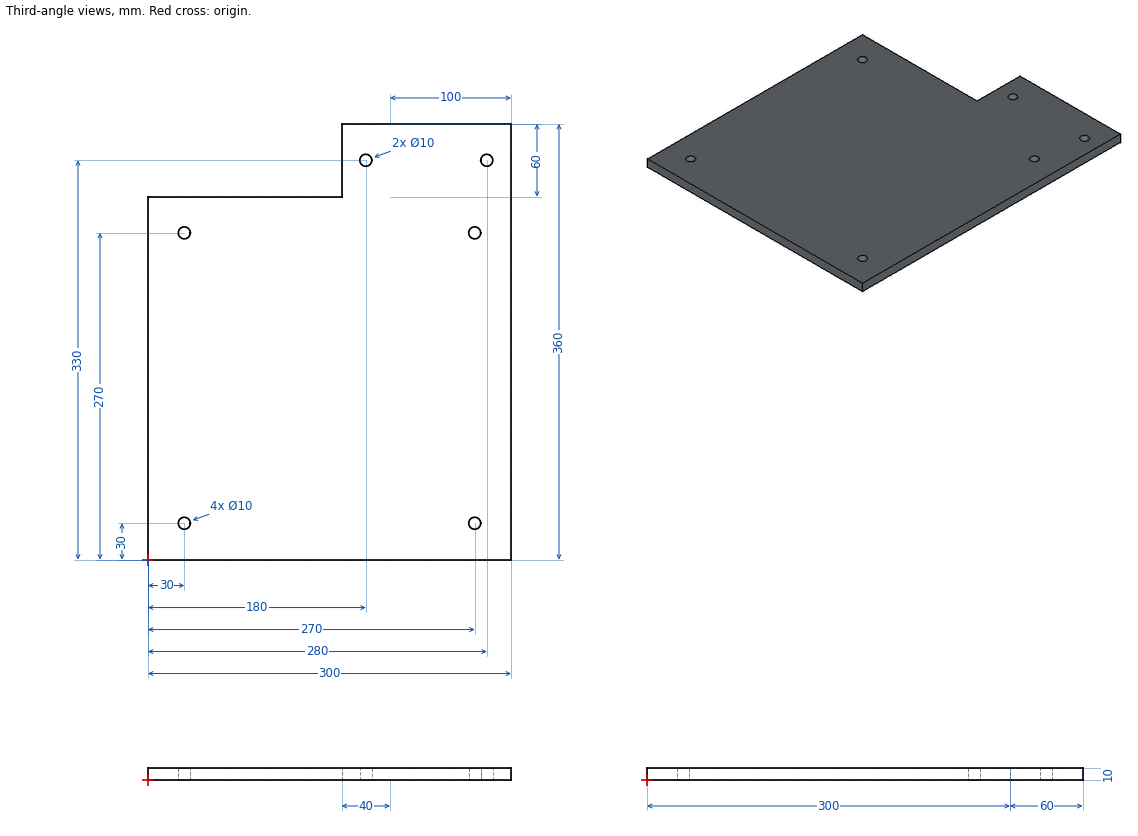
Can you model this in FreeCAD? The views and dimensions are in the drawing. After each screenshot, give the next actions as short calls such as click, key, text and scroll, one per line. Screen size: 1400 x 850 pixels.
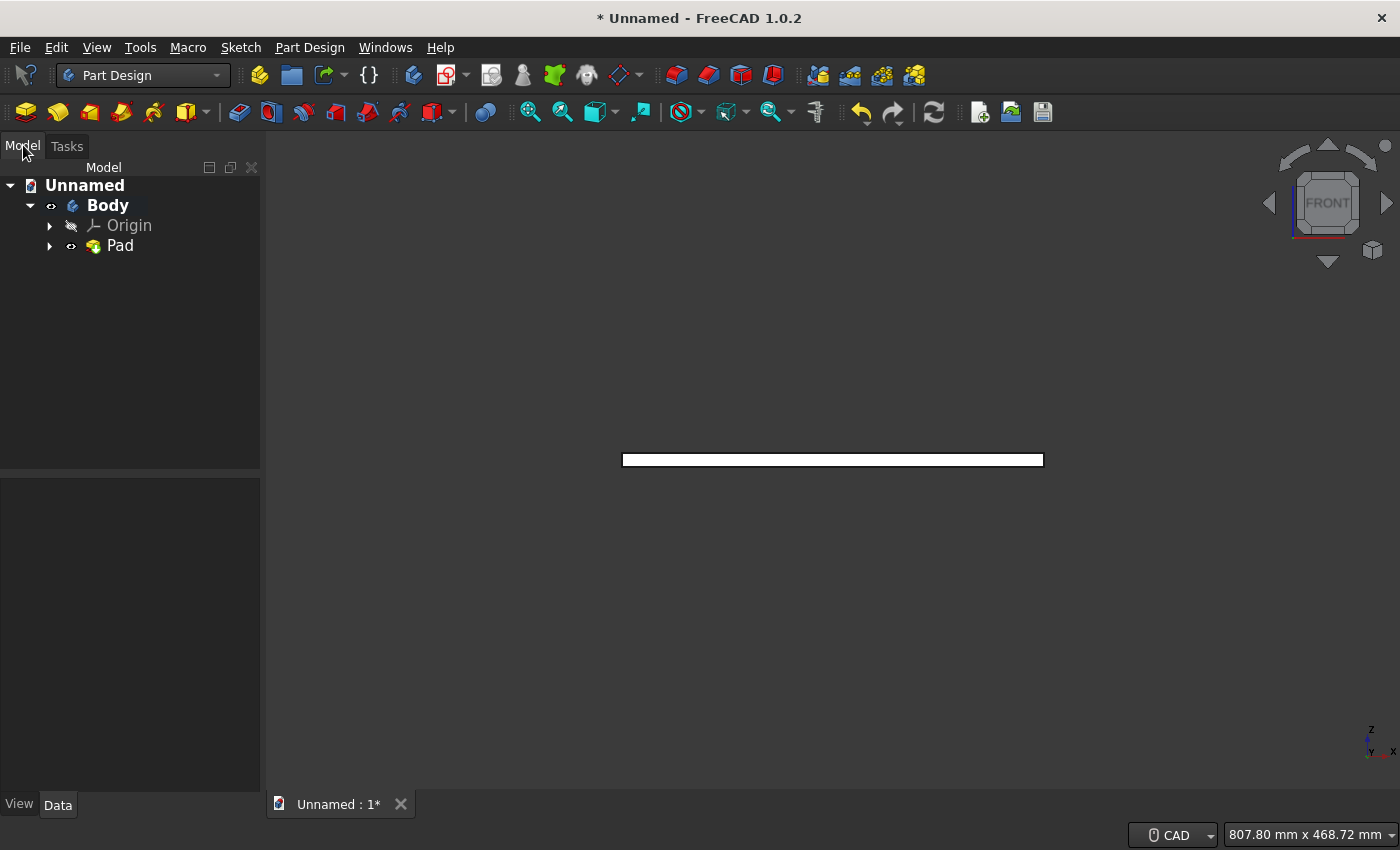
click(50, 226)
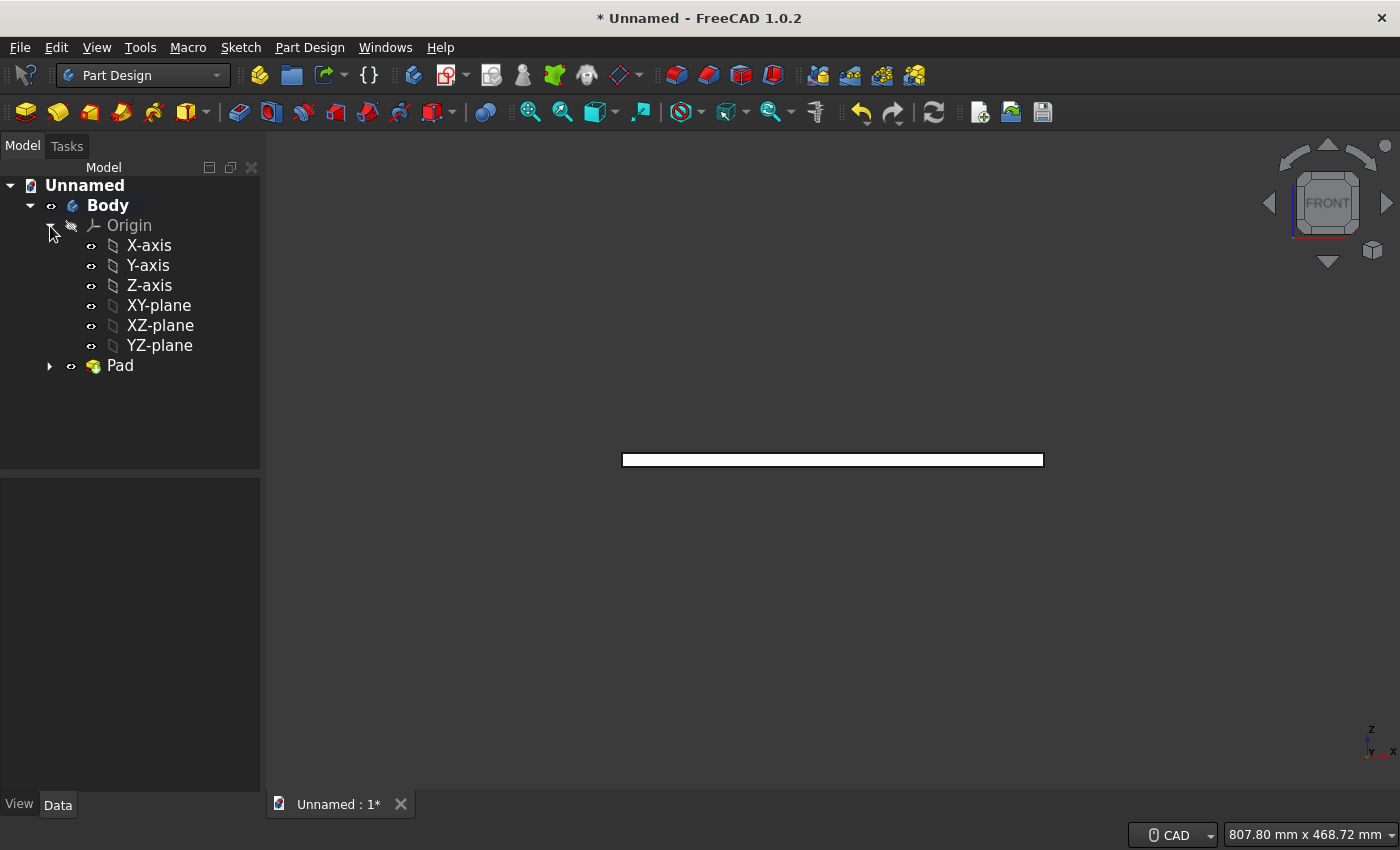
click(136, 346)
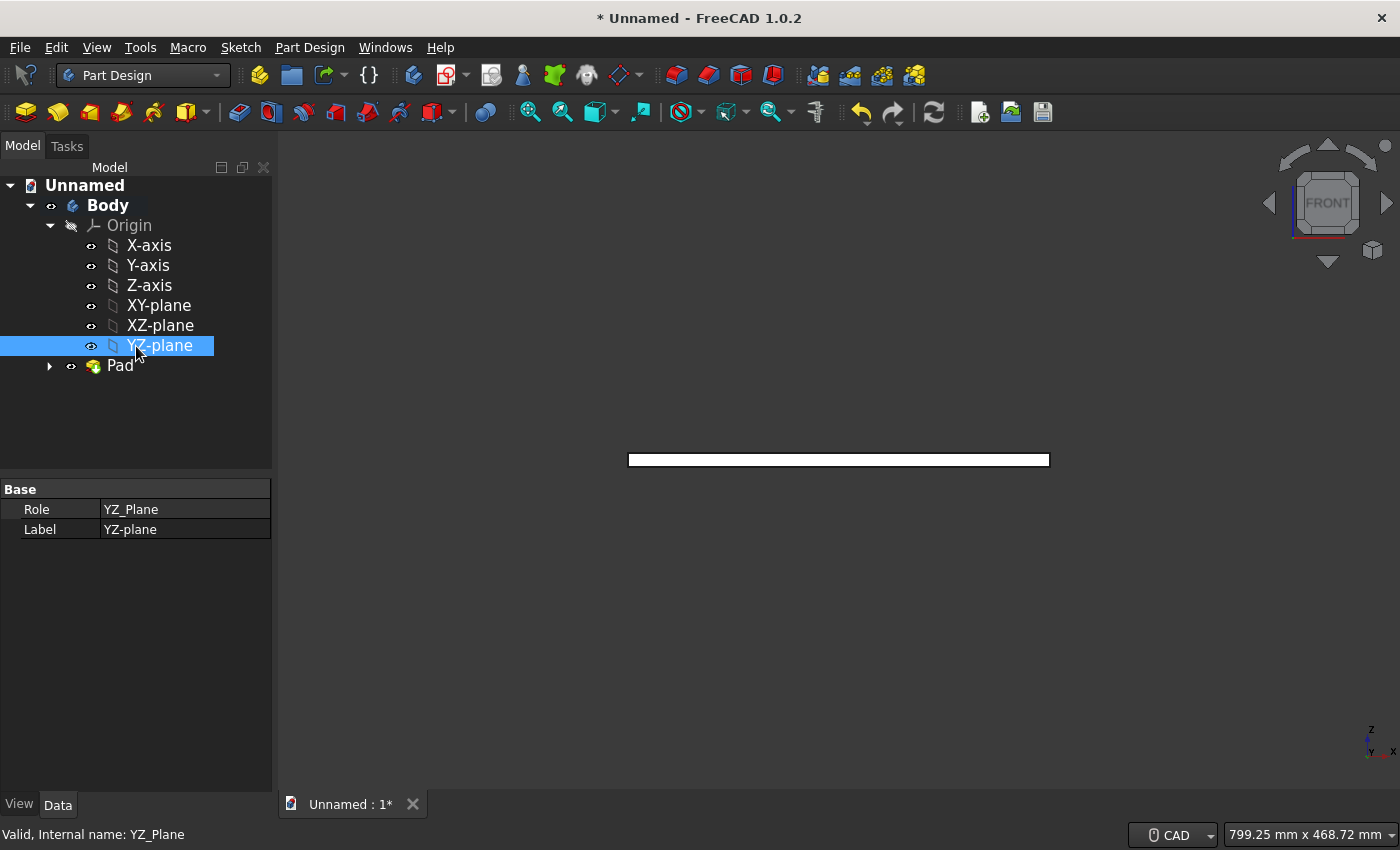
click(620, 76)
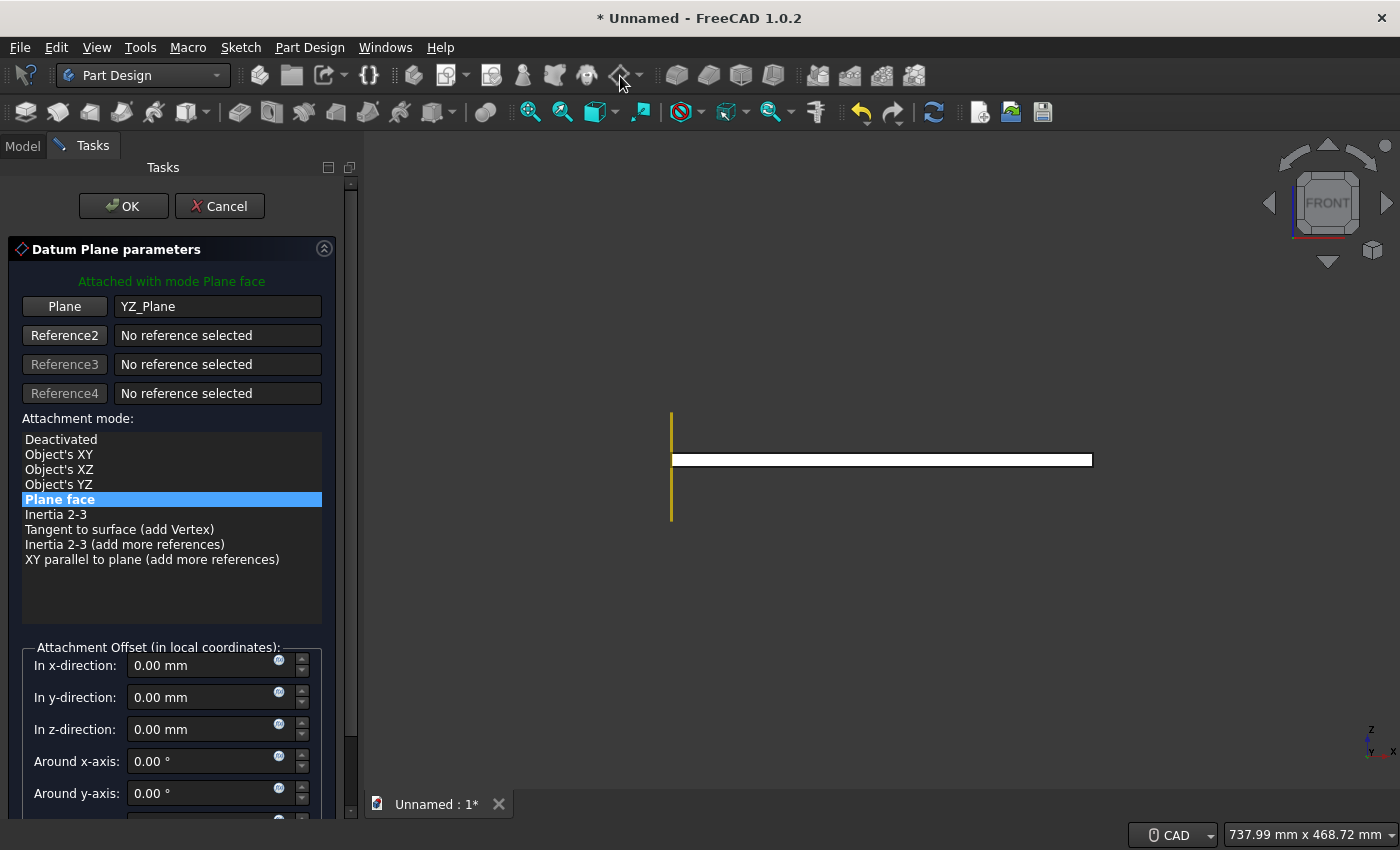
triple_click(210, 729)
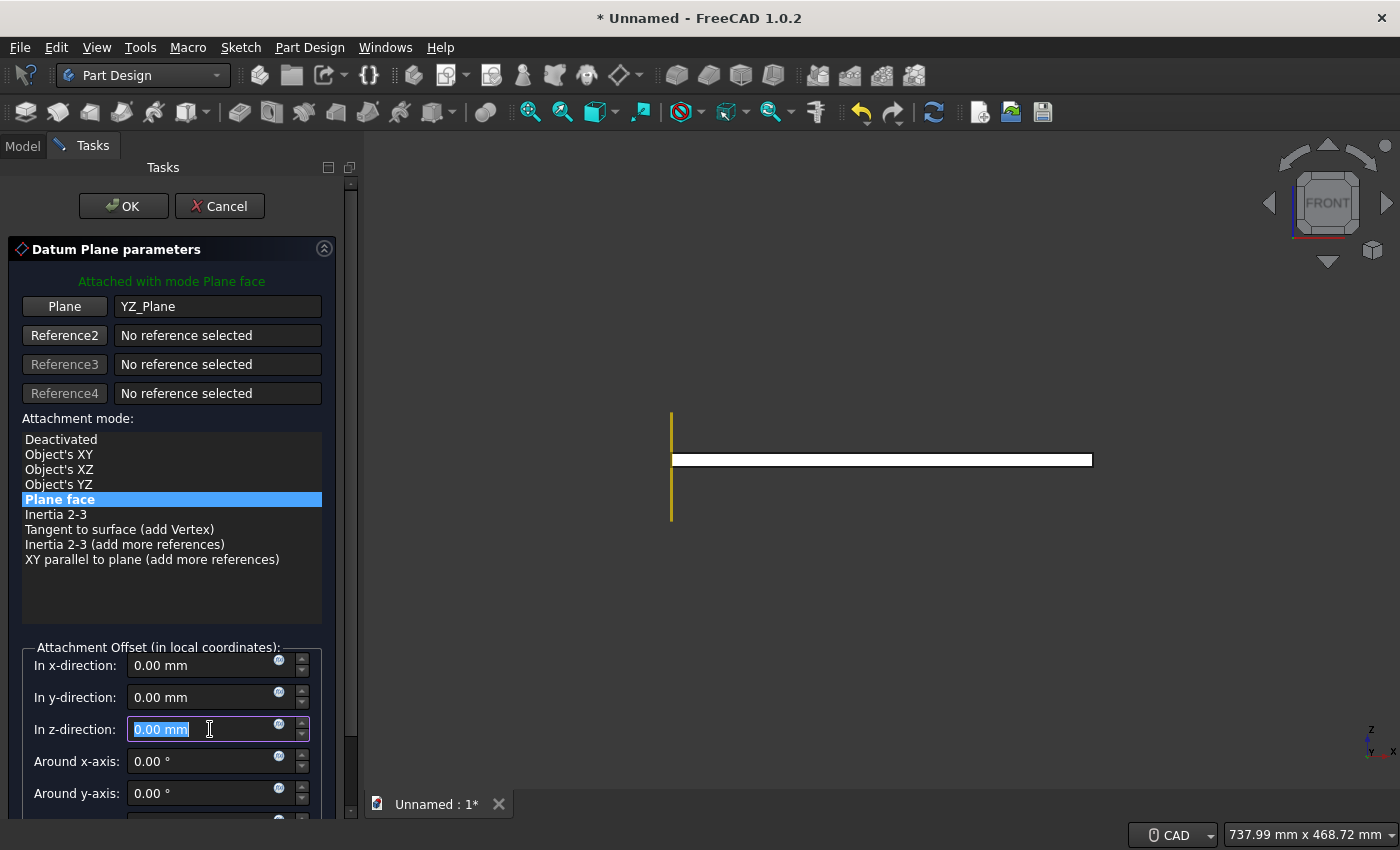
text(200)
key(Tab)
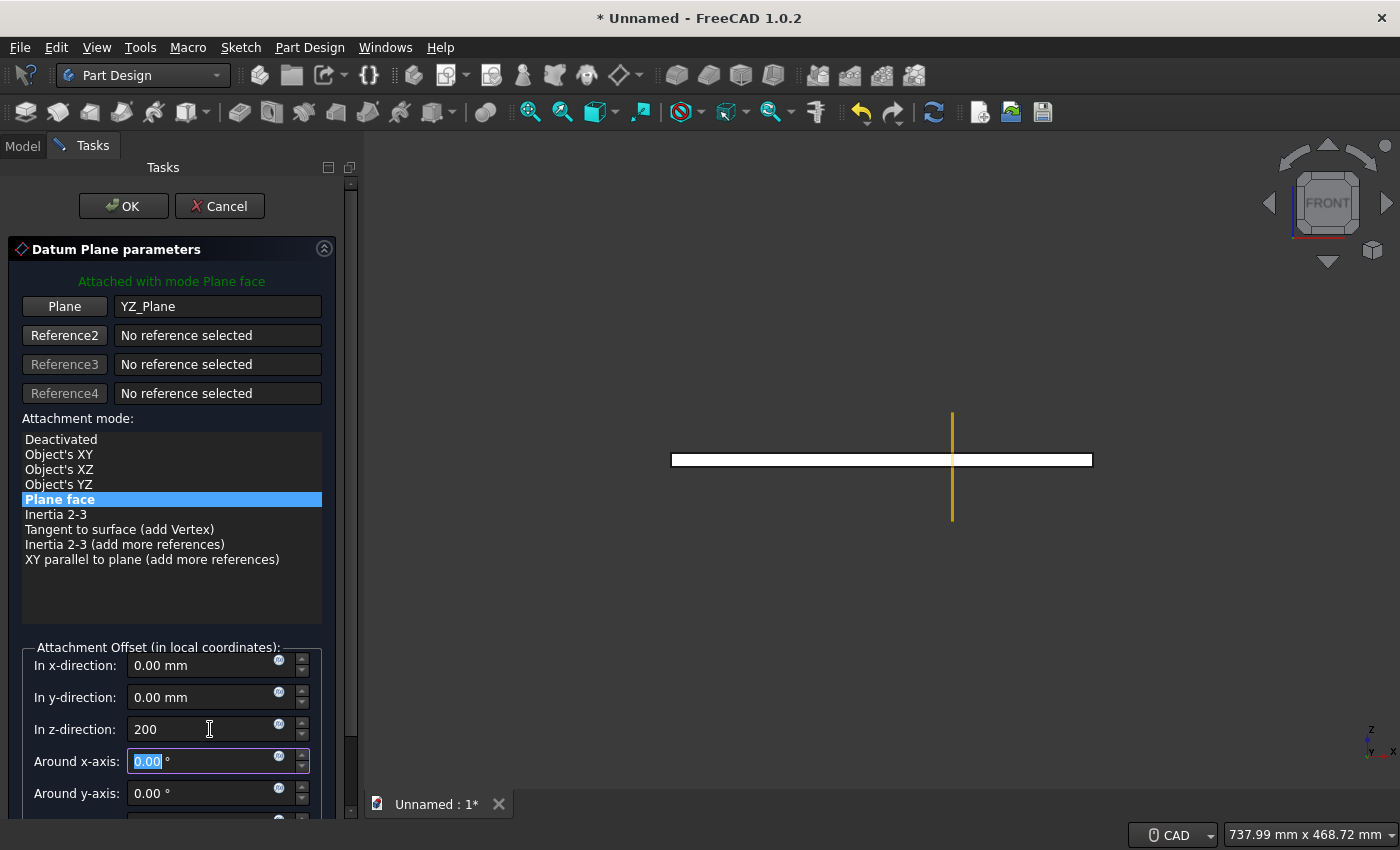
click(124, 206)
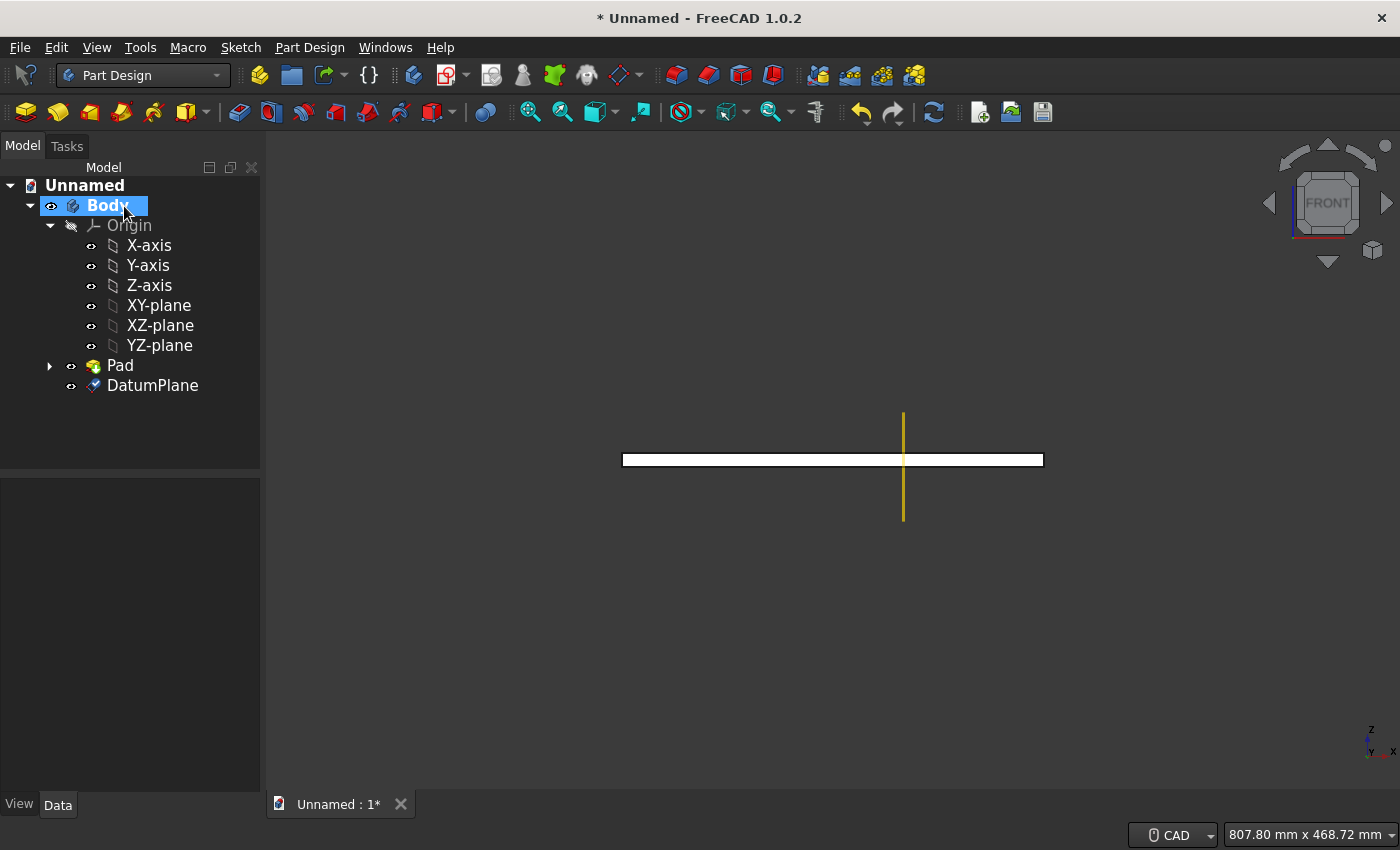
click(116, 386)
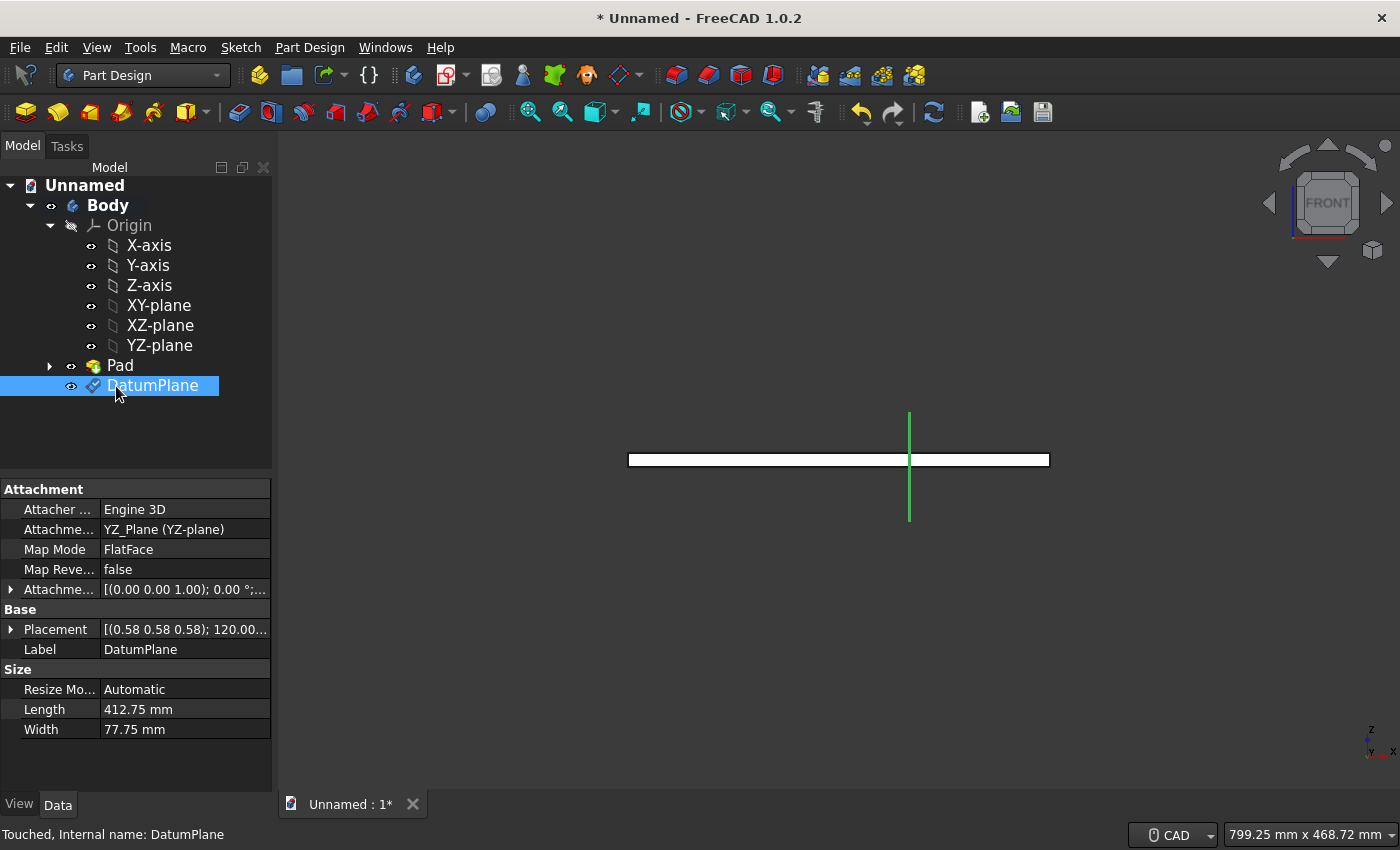
click(446, 76)